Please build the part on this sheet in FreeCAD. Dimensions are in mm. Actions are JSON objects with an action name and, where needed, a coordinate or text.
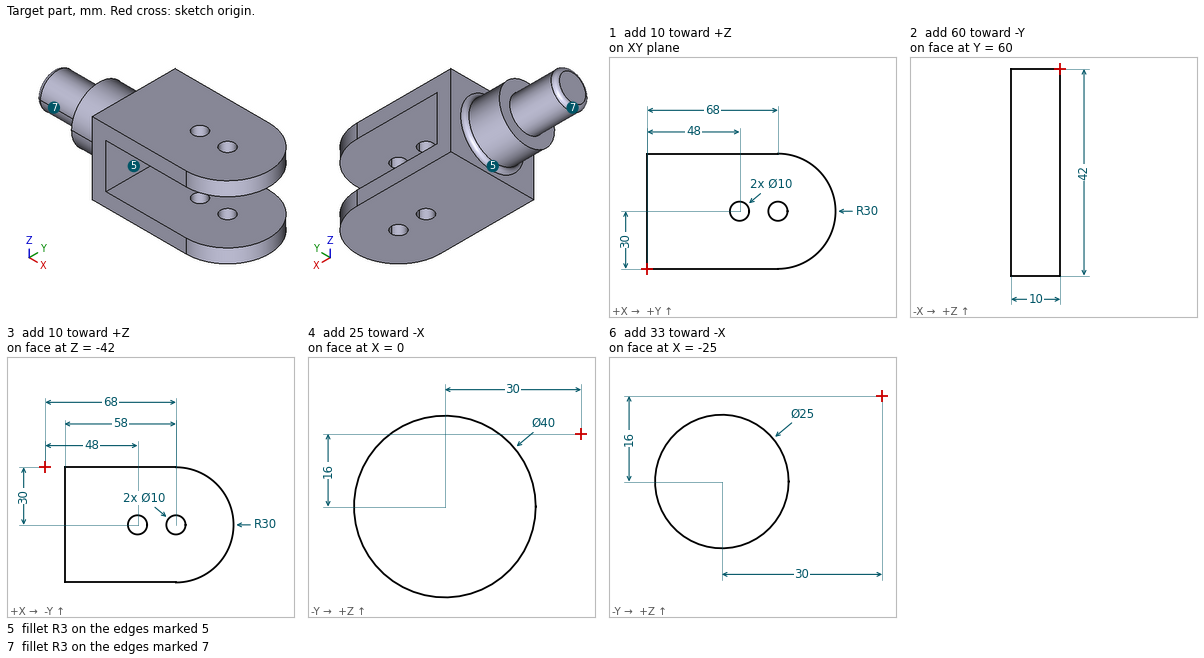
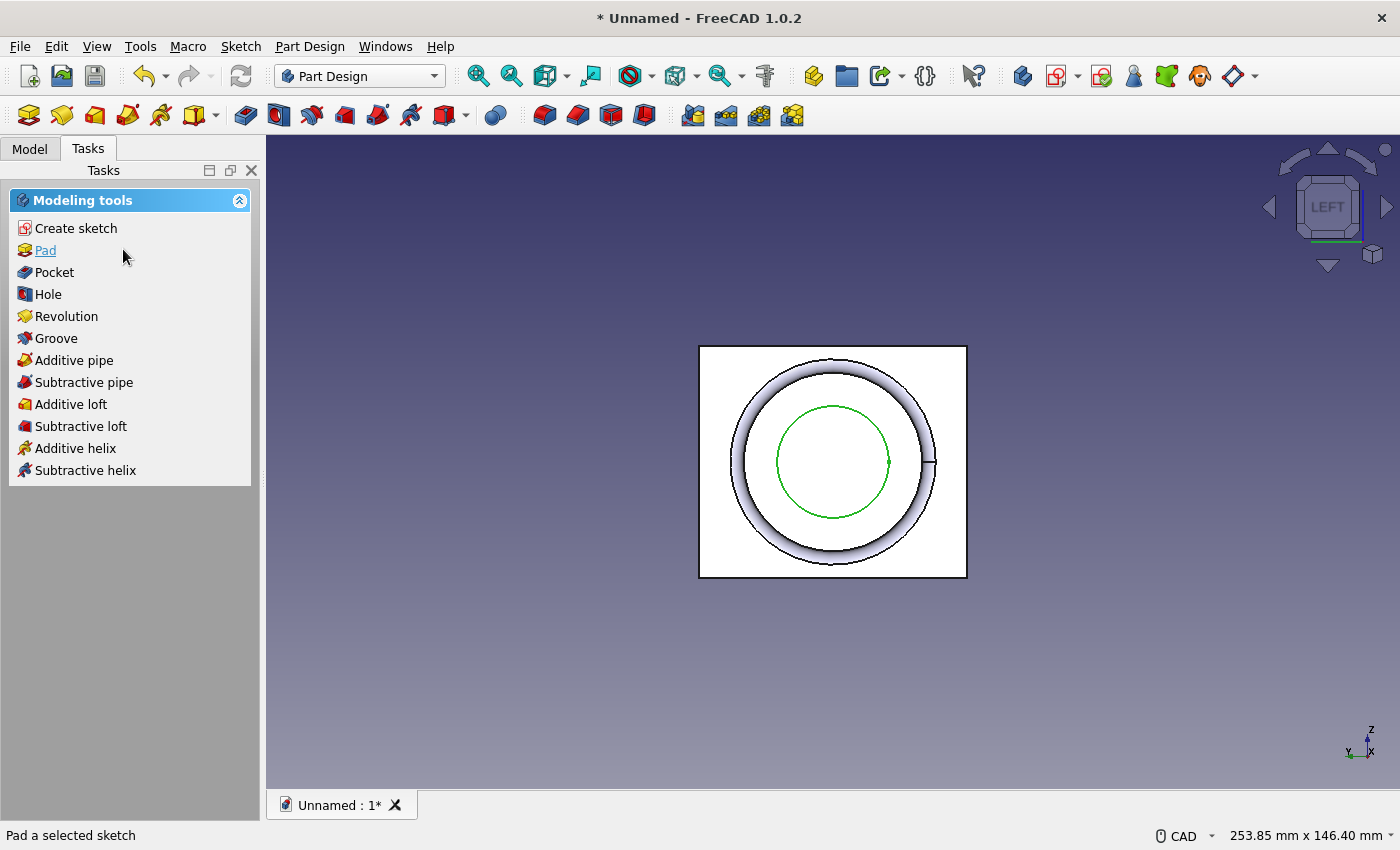
{"action": "left_click", "coordinate": [29, 116]}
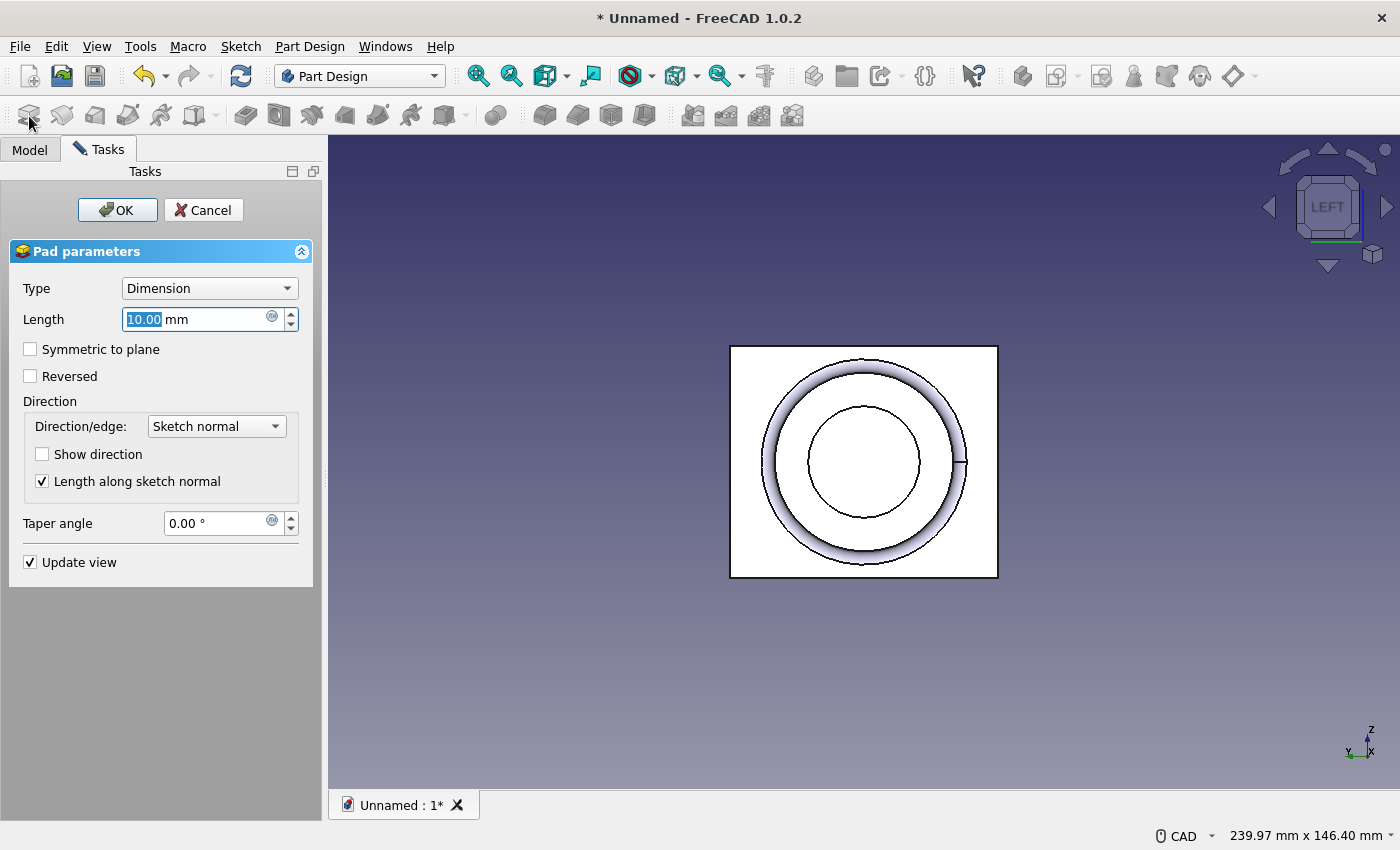
{"action": "type", "text": "33"}
{"action": "key", "text": "Tab"}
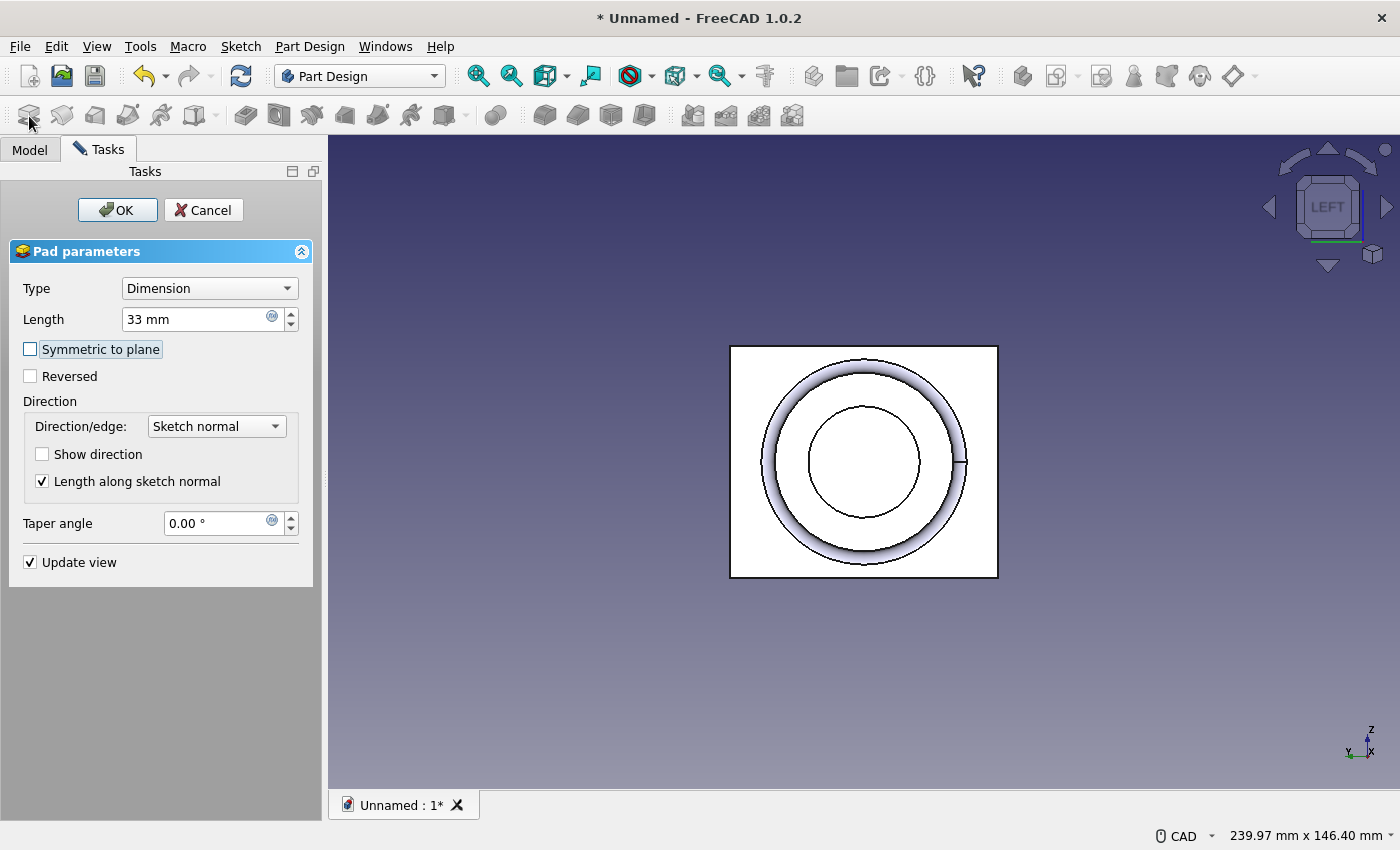
{"action": "left_click", "coordinate": [118, 210]}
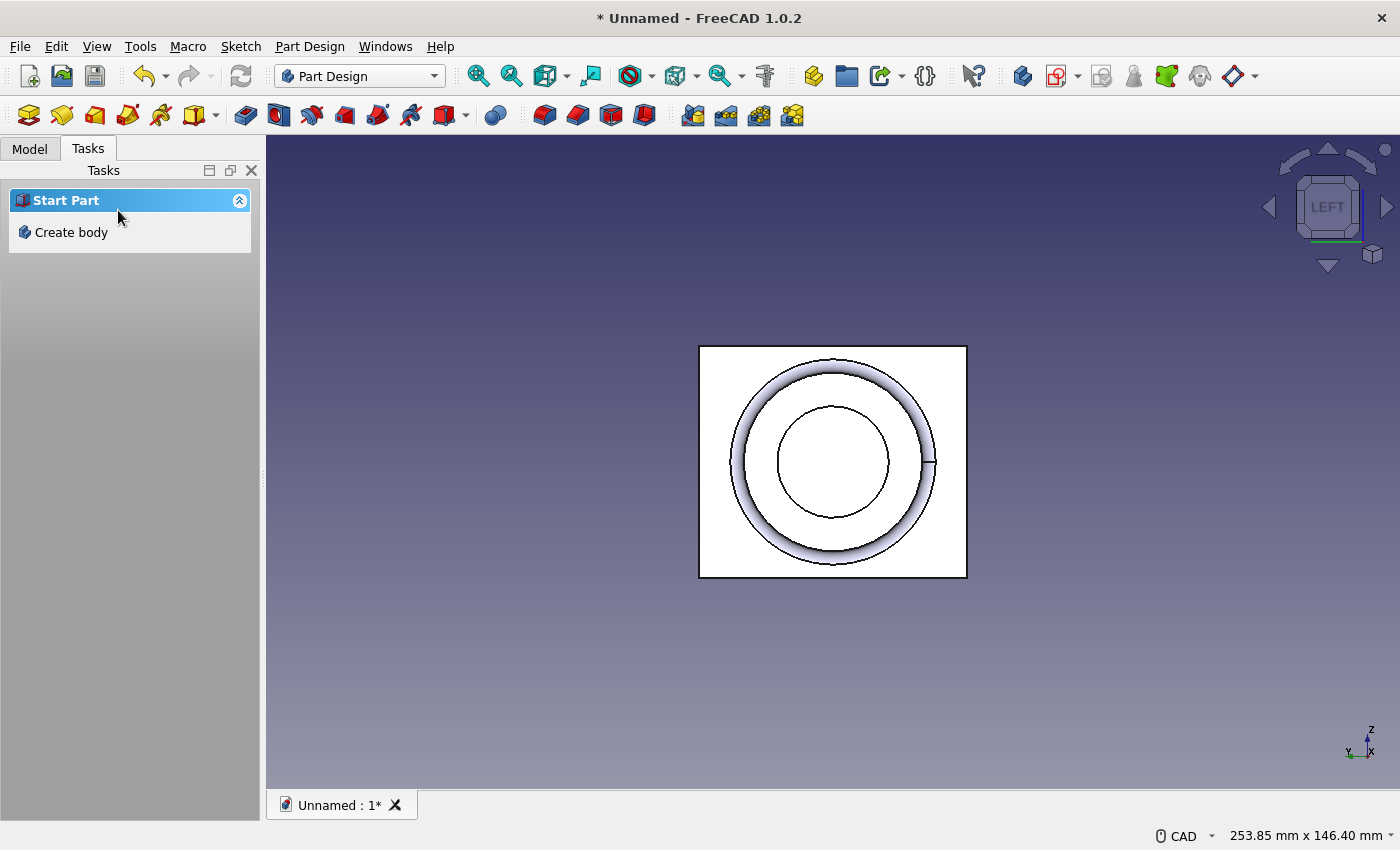
{"action": "key", "text": "v f"}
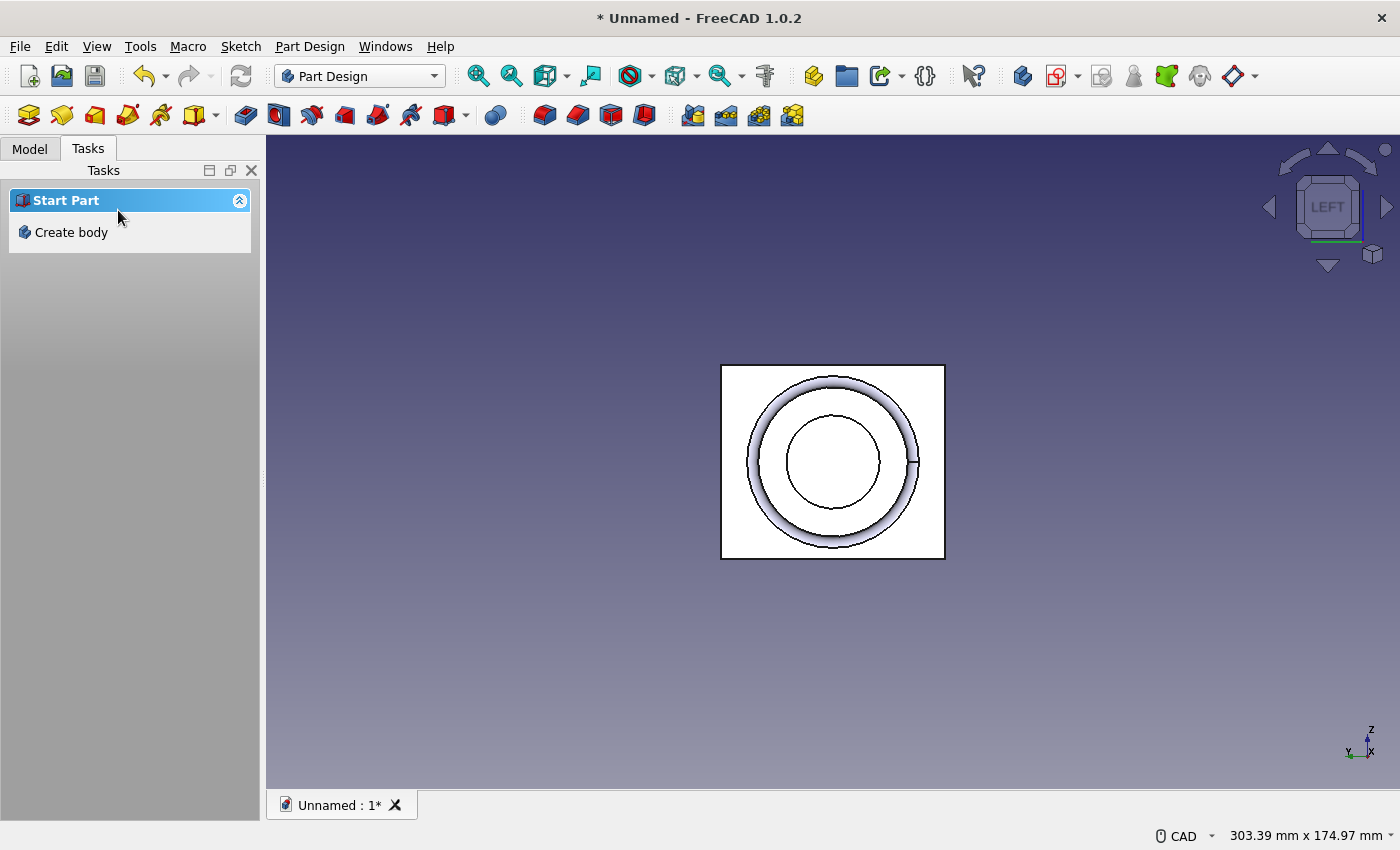
{"action": "left_click", "coordinate": [786, 461]}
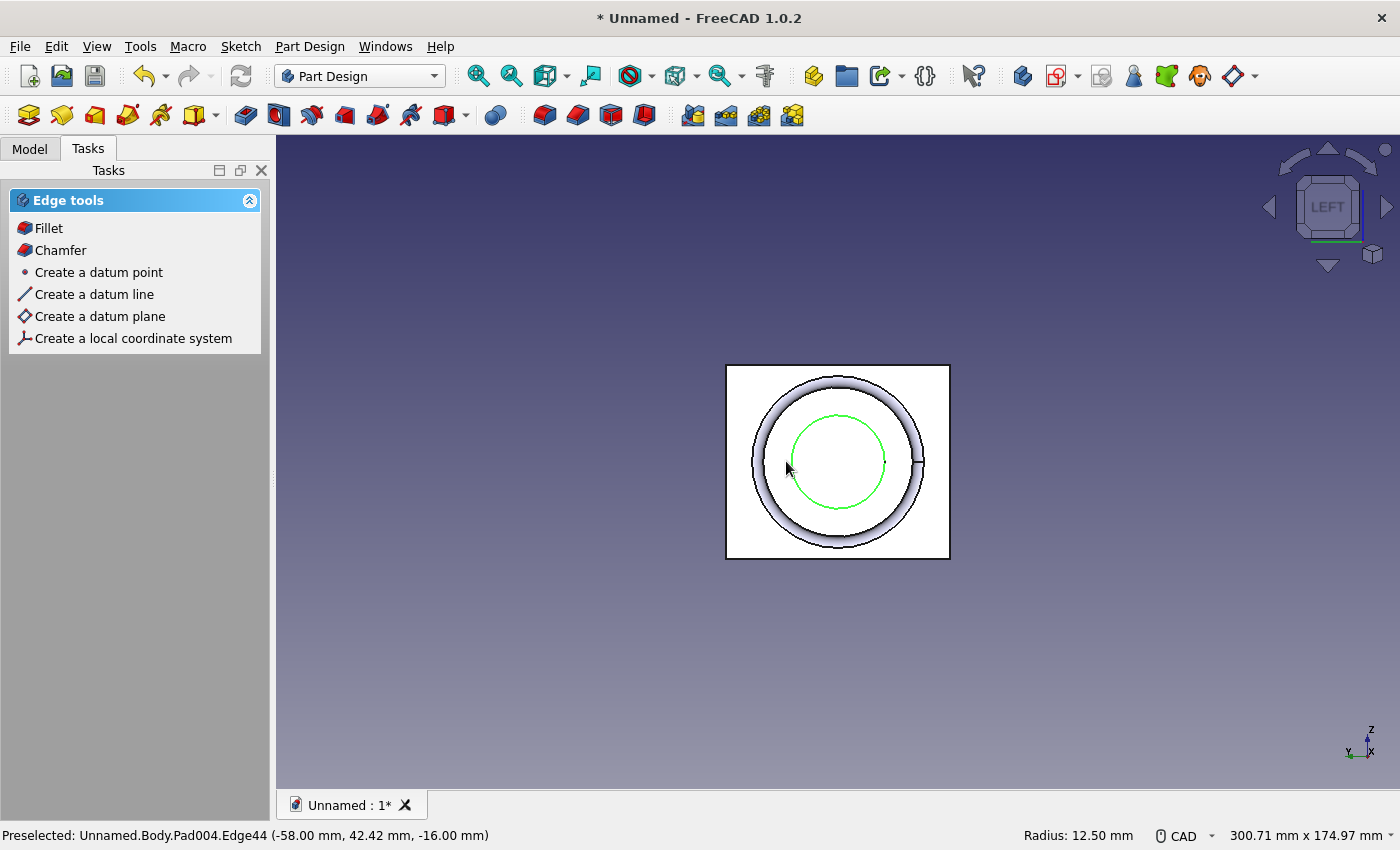
{"action": "left_click", "coordinate": [545, 116]}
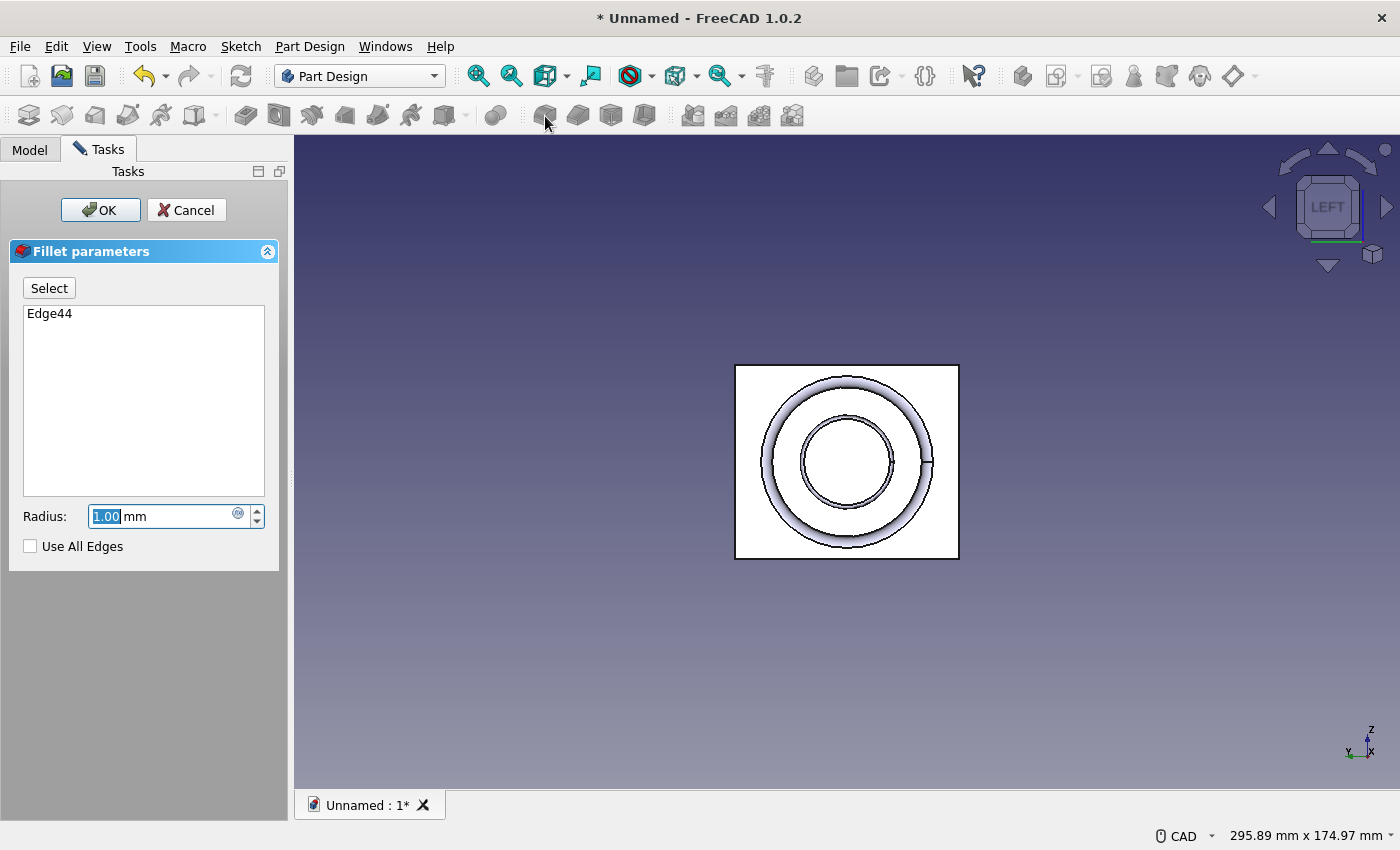
{"action": "type", "text": "3"}
{"action": "key", "text": "Tab"}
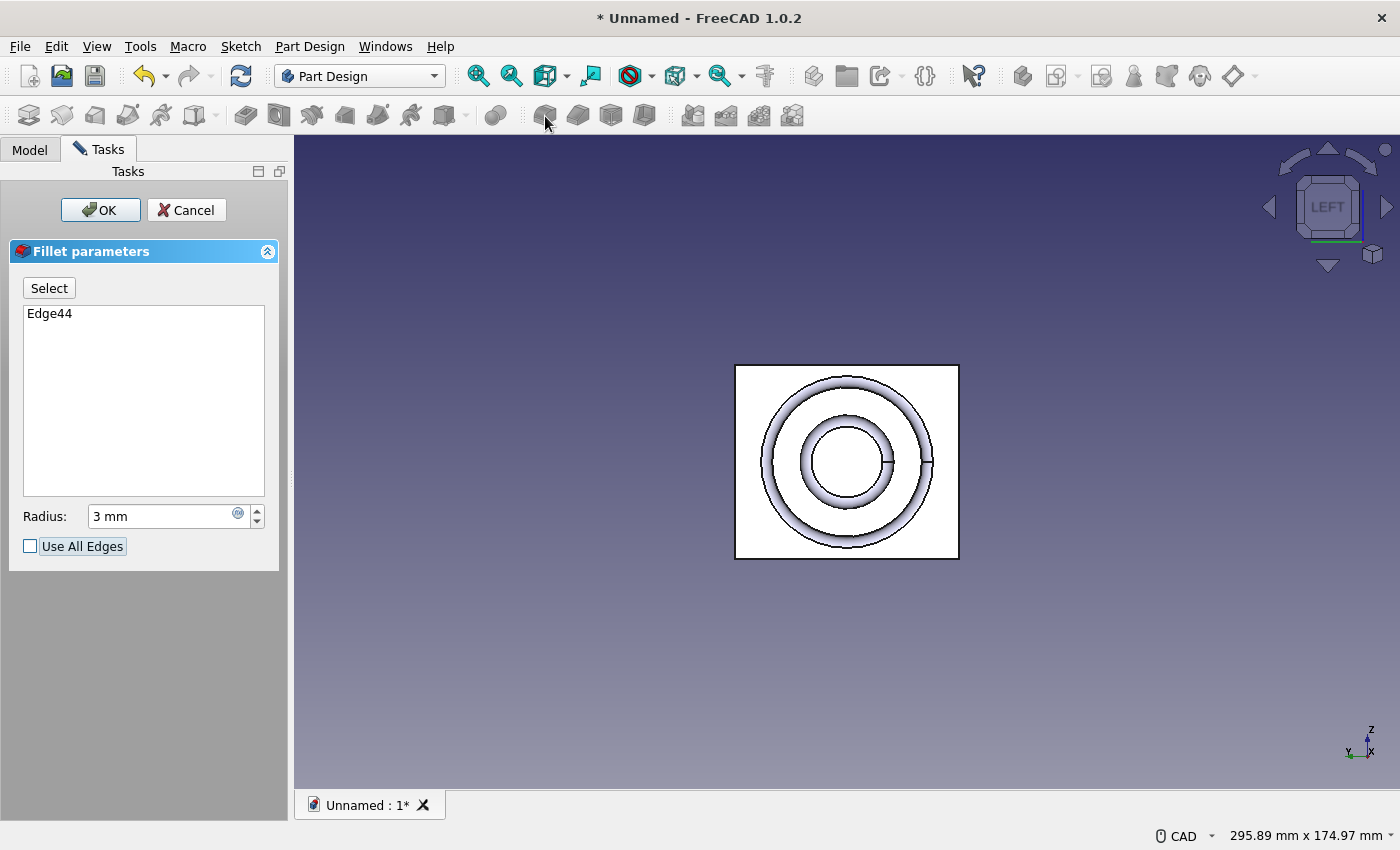
{"action": "left_click", "coordinate": [101, 210]}